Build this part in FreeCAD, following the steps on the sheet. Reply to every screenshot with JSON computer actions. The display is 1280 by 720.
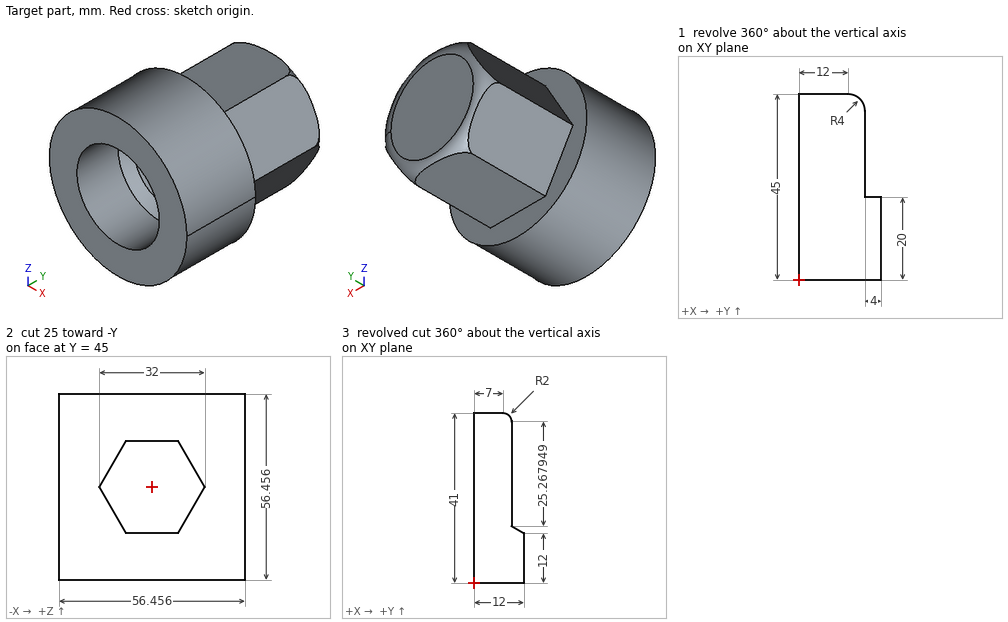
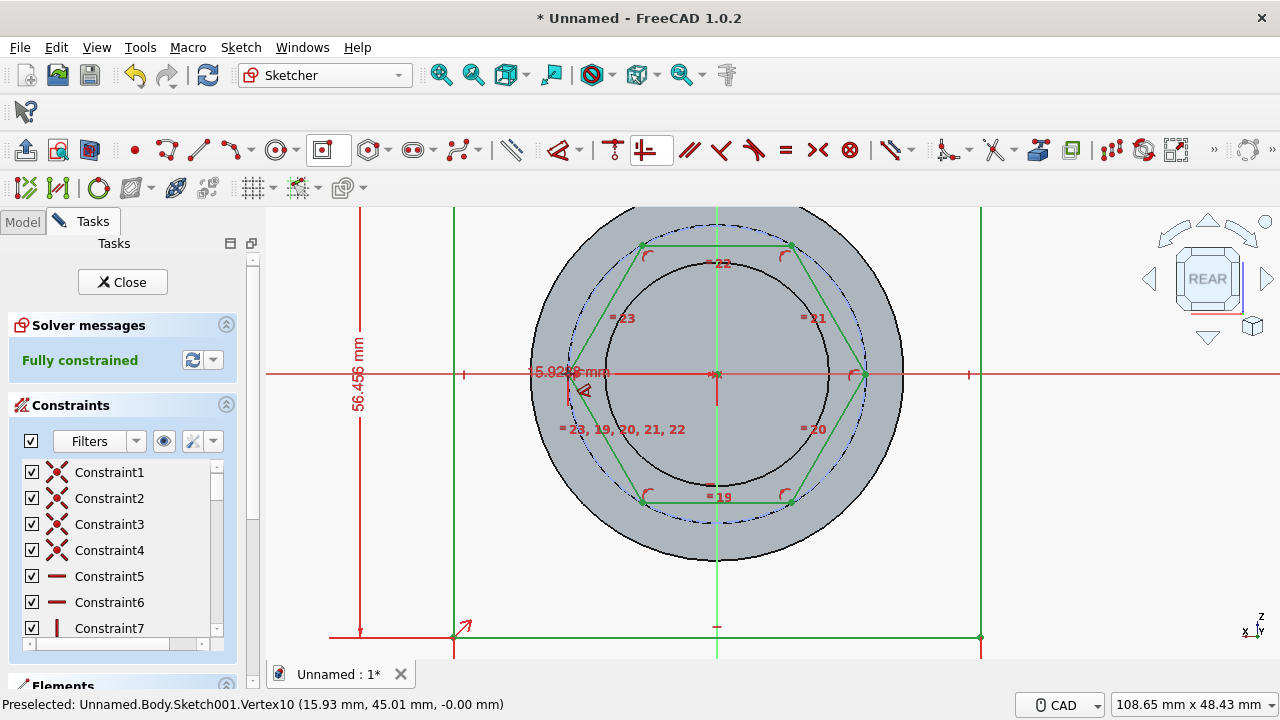
{"action": "left_click", "coordinate": [866, 374]}
{"action": "left_click", "coordinate": [649, 408]}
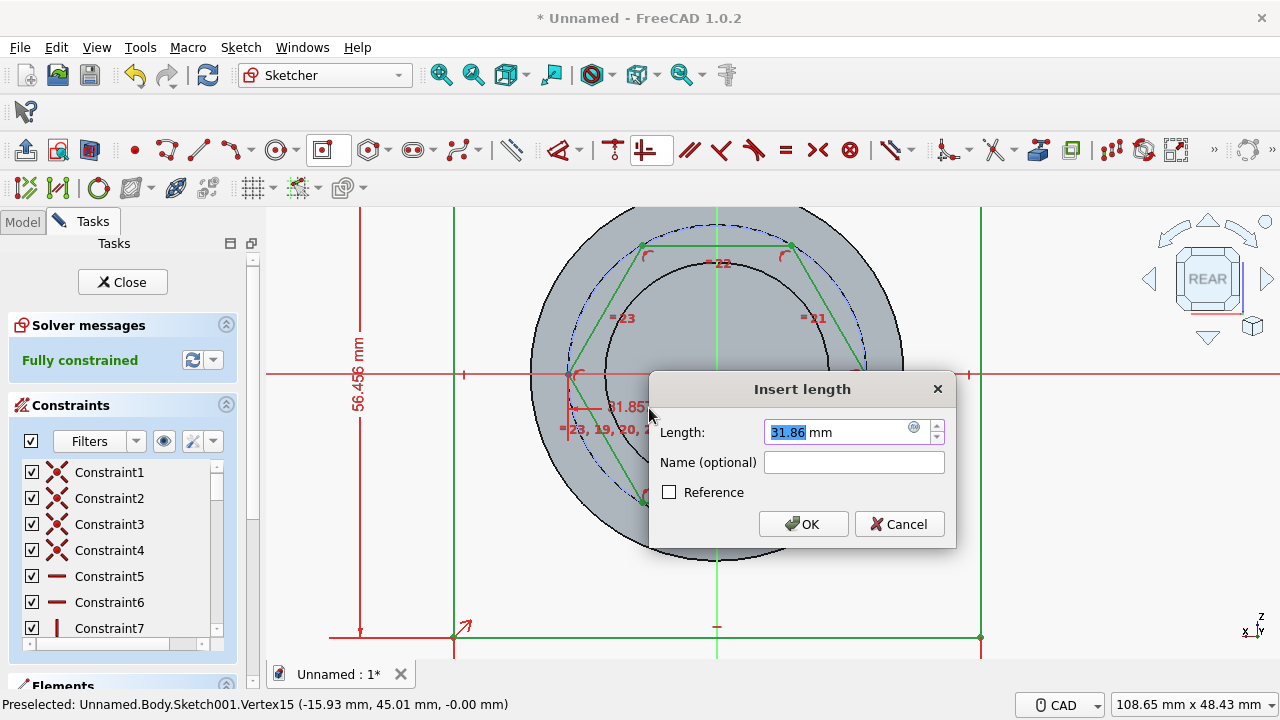
{"action": "type", "text": "32"}
{"action": "key", "text": "Return"}
{"action": "key", "text": "Escape"}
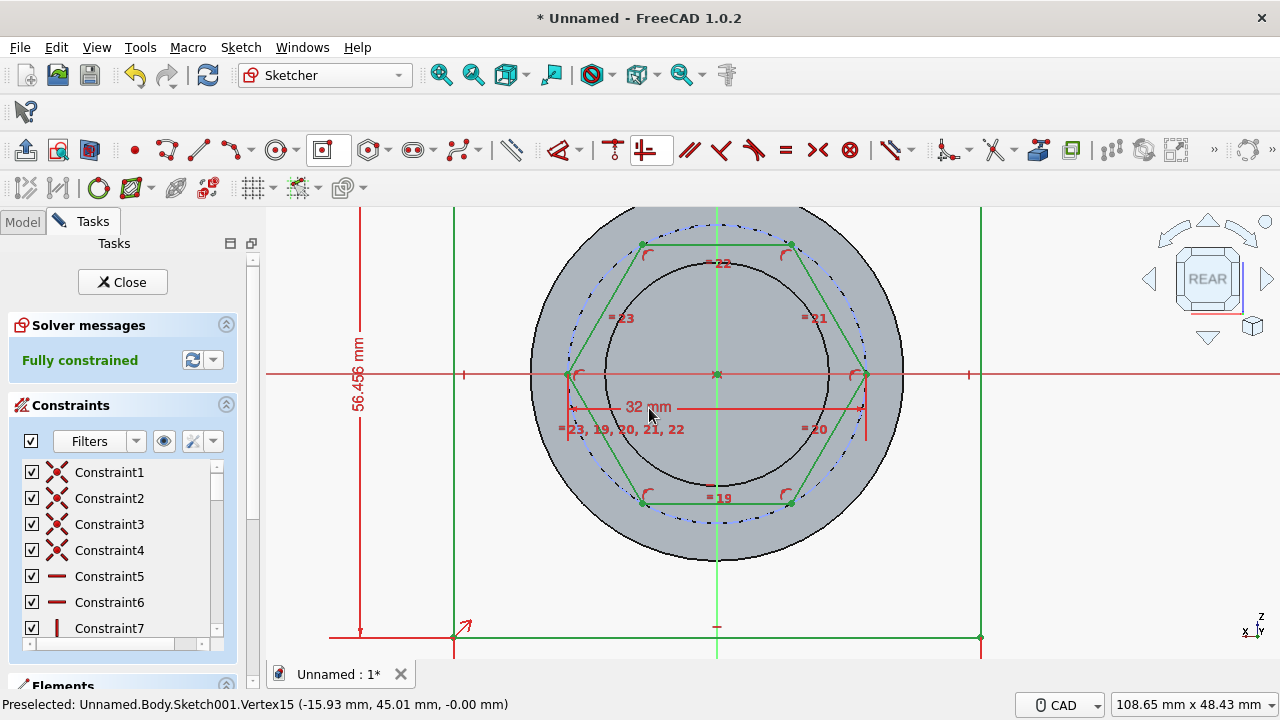
{"action": "left_click", "coordinate": [123, 282]}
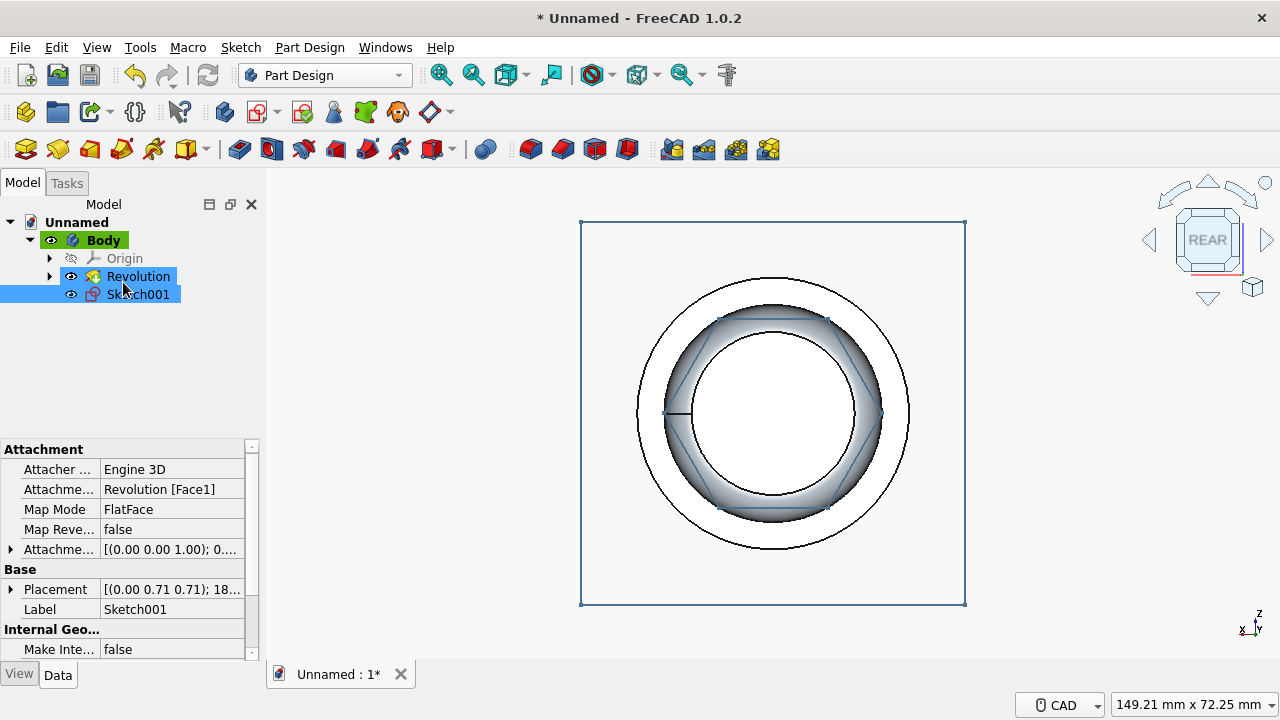
{"action": "left_click", "coordinate": [240, 150]}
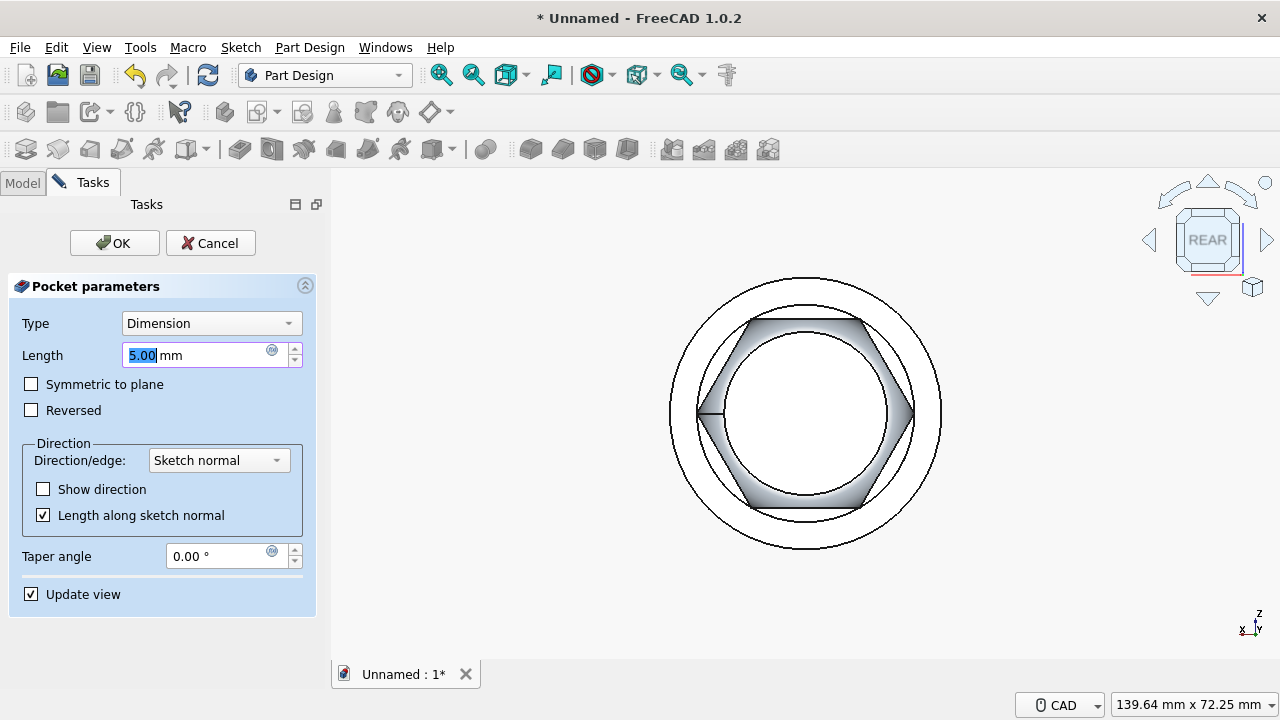
{"action": "type", "text": "25"}
{"action": "key", "text": "Tab"}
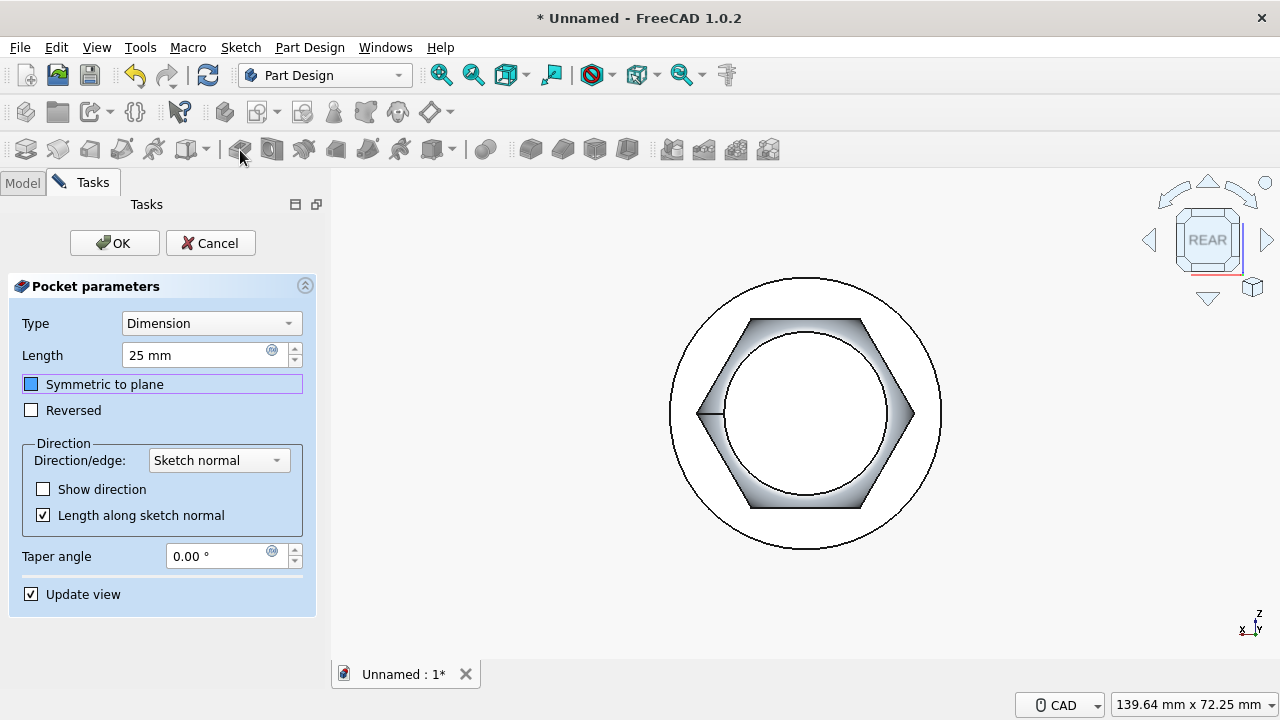
{"action": "left_click", "coordinate": [115, 243]}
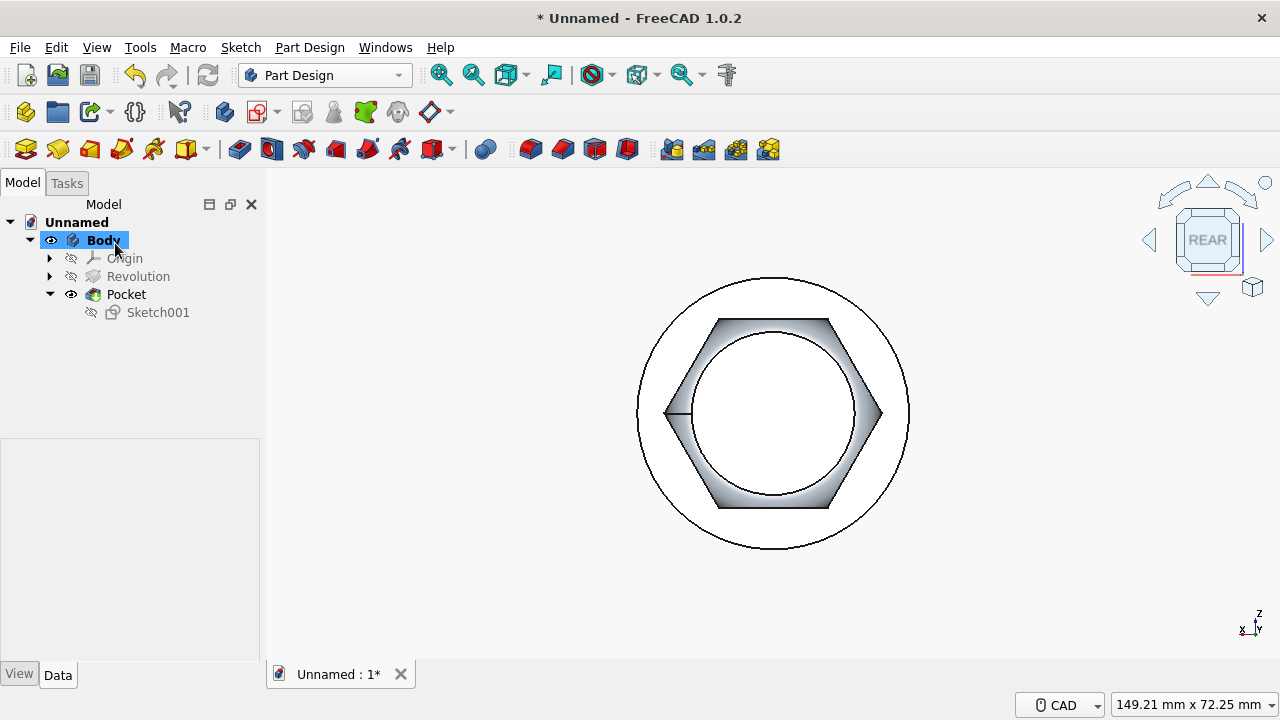
{"action": "left_click", "coordinate": [258, 112]}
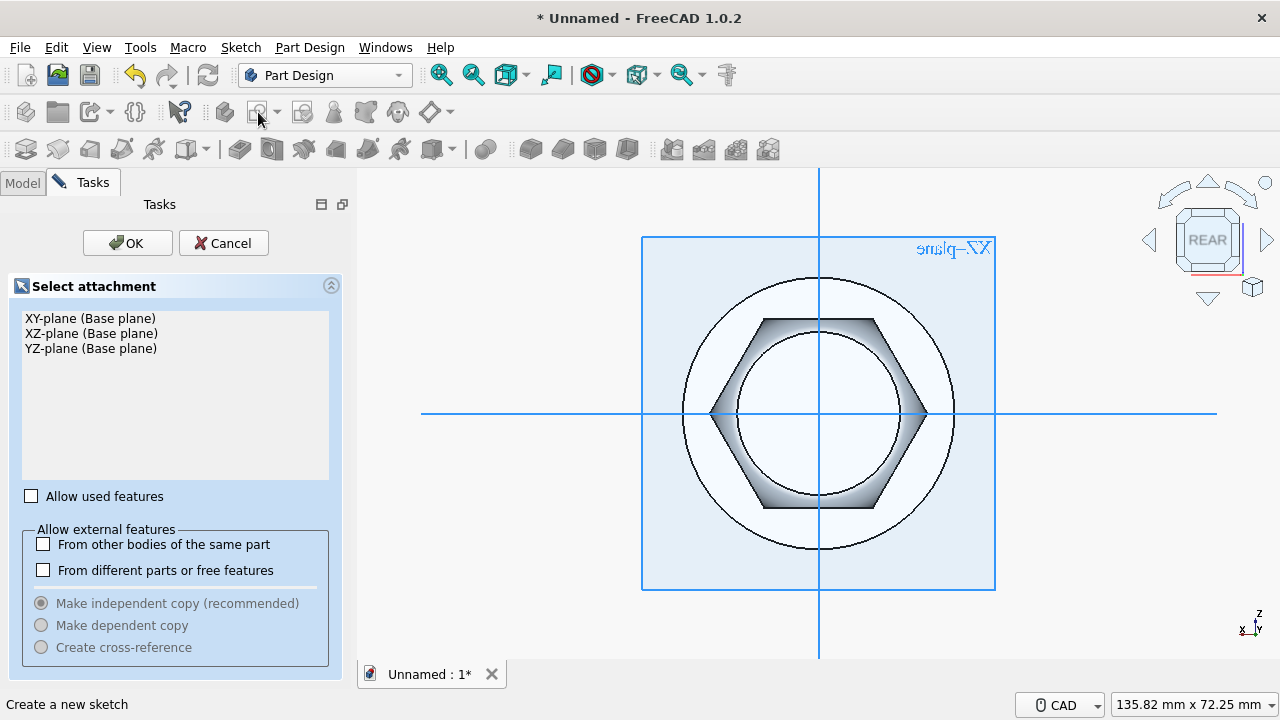
{"action": "left_click", "coordinate": [82, 318]}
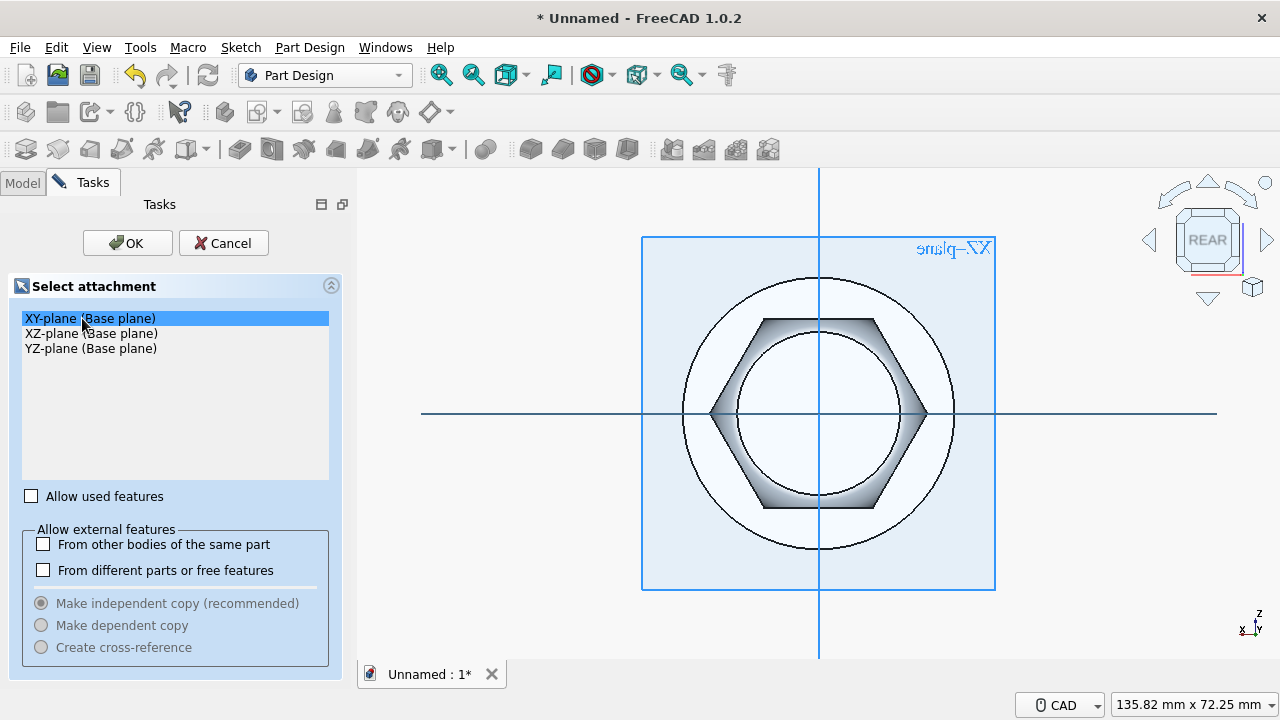
{"action": "left_click", "coordinate": [128, 243]}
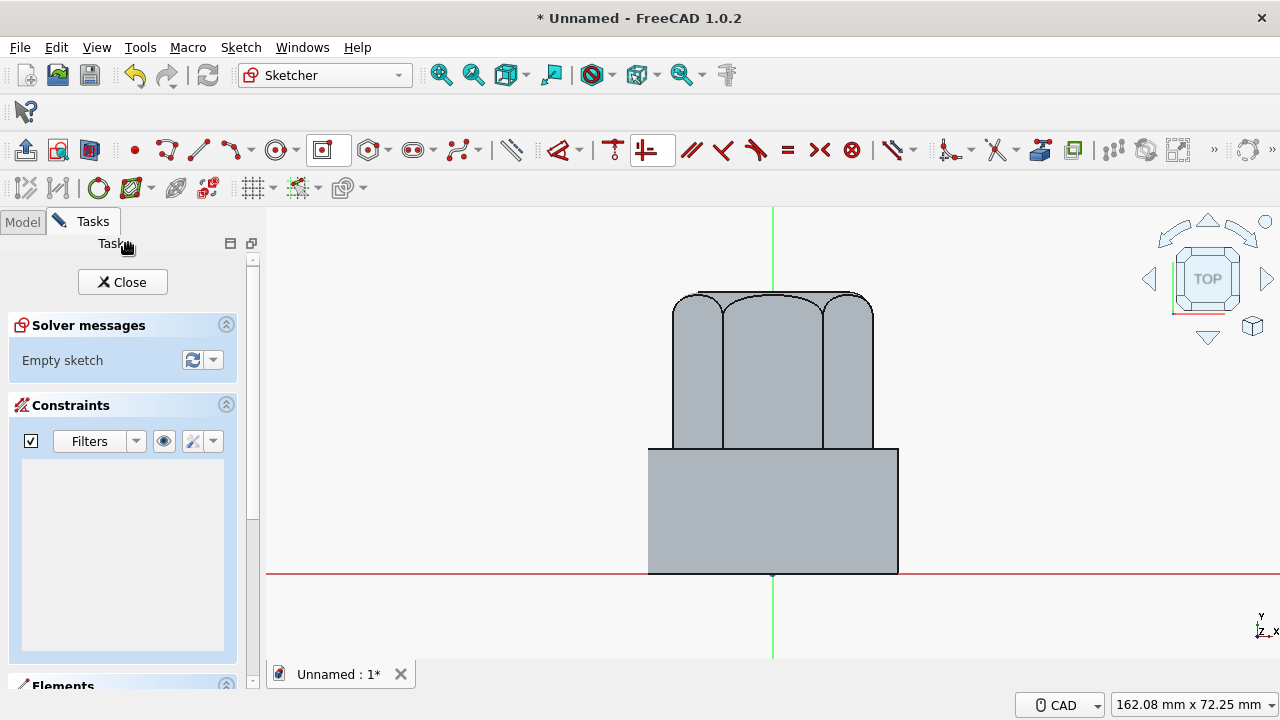
{"action": "key", "text": "q s"}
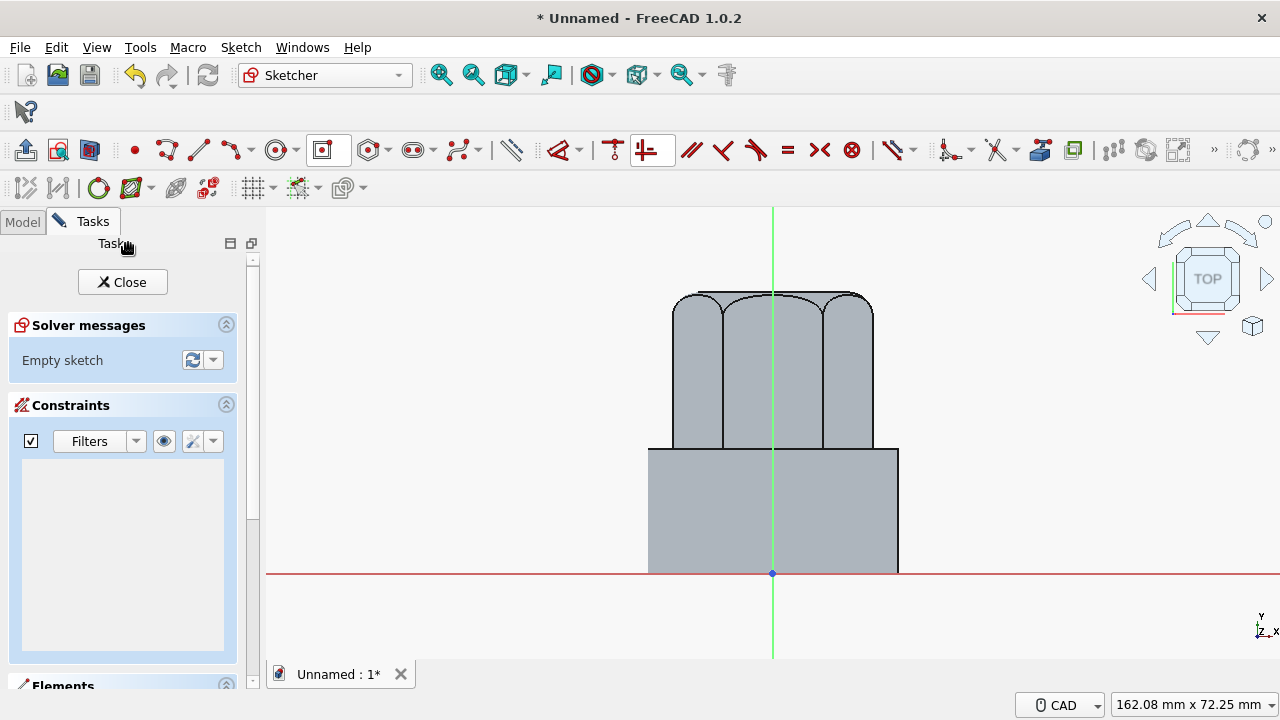
{"action": "key", "text": "g m"}